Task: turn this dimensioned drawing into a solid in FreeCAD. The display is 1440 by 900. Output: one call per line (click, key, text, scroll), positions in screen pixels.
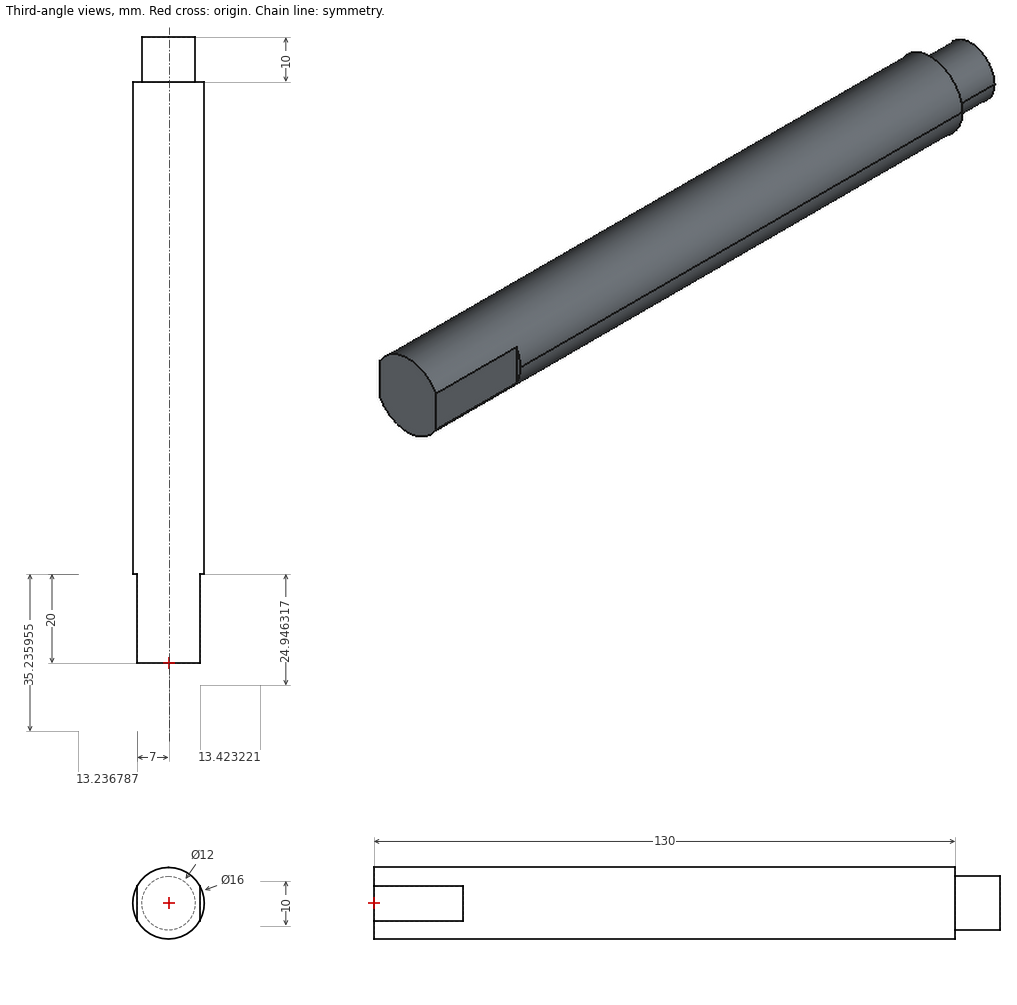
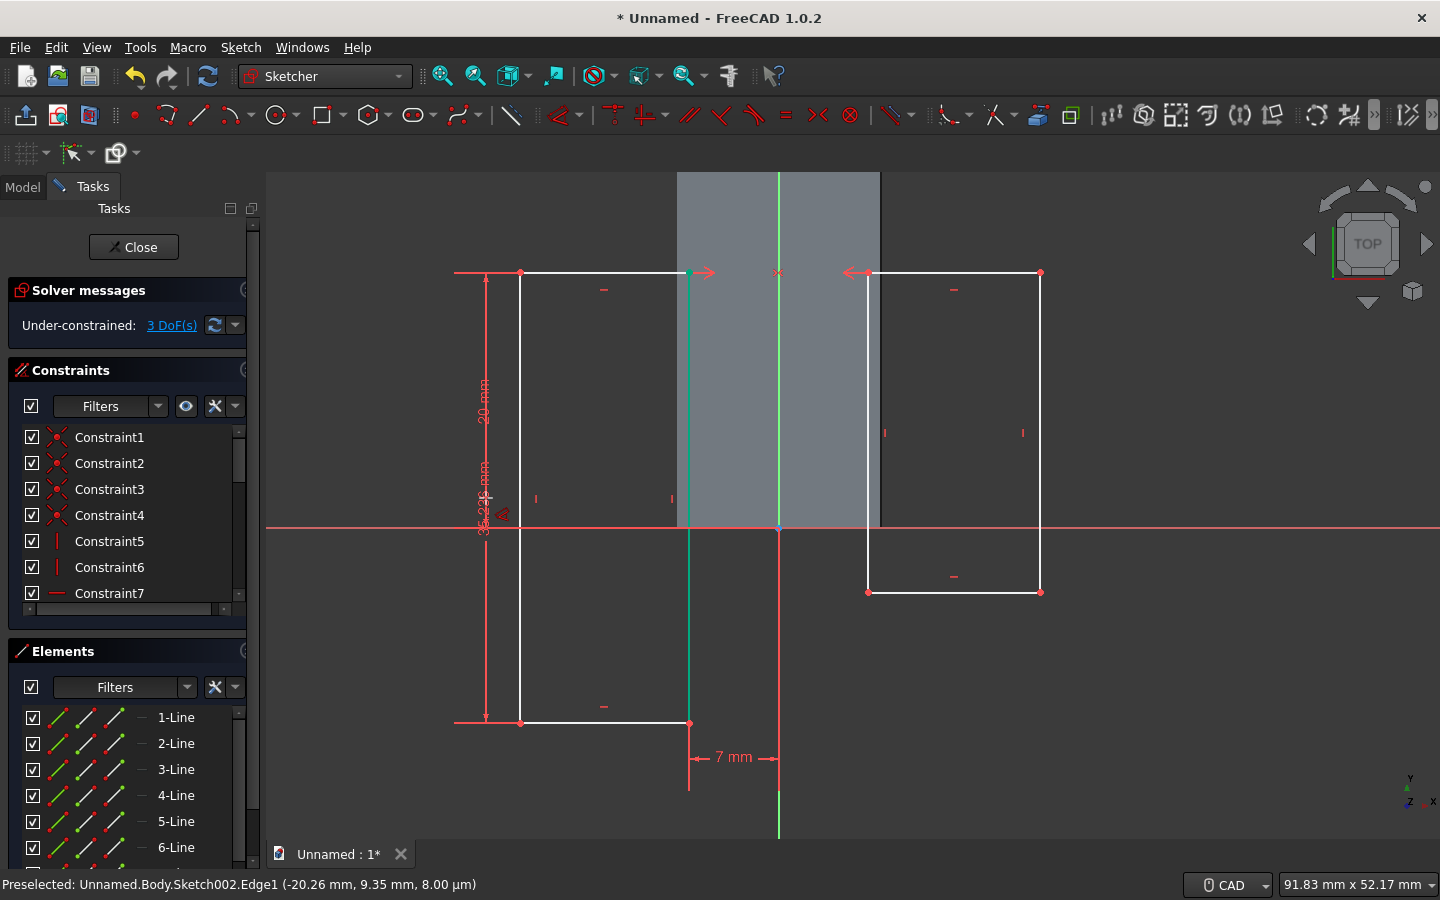
click(571, 723)
click(605, 757)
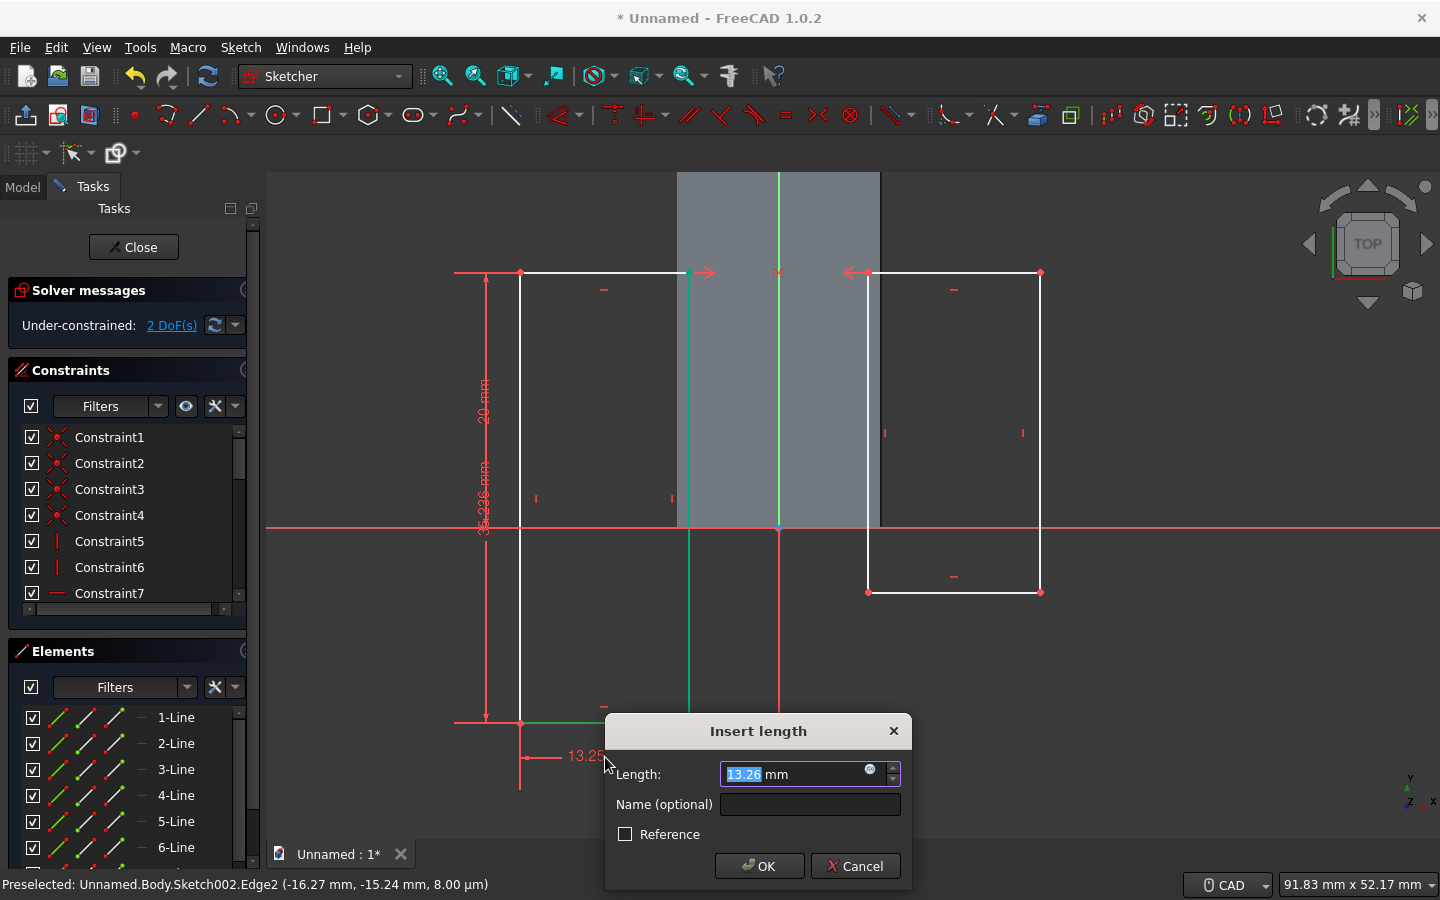
text(13.236787)
key(Return)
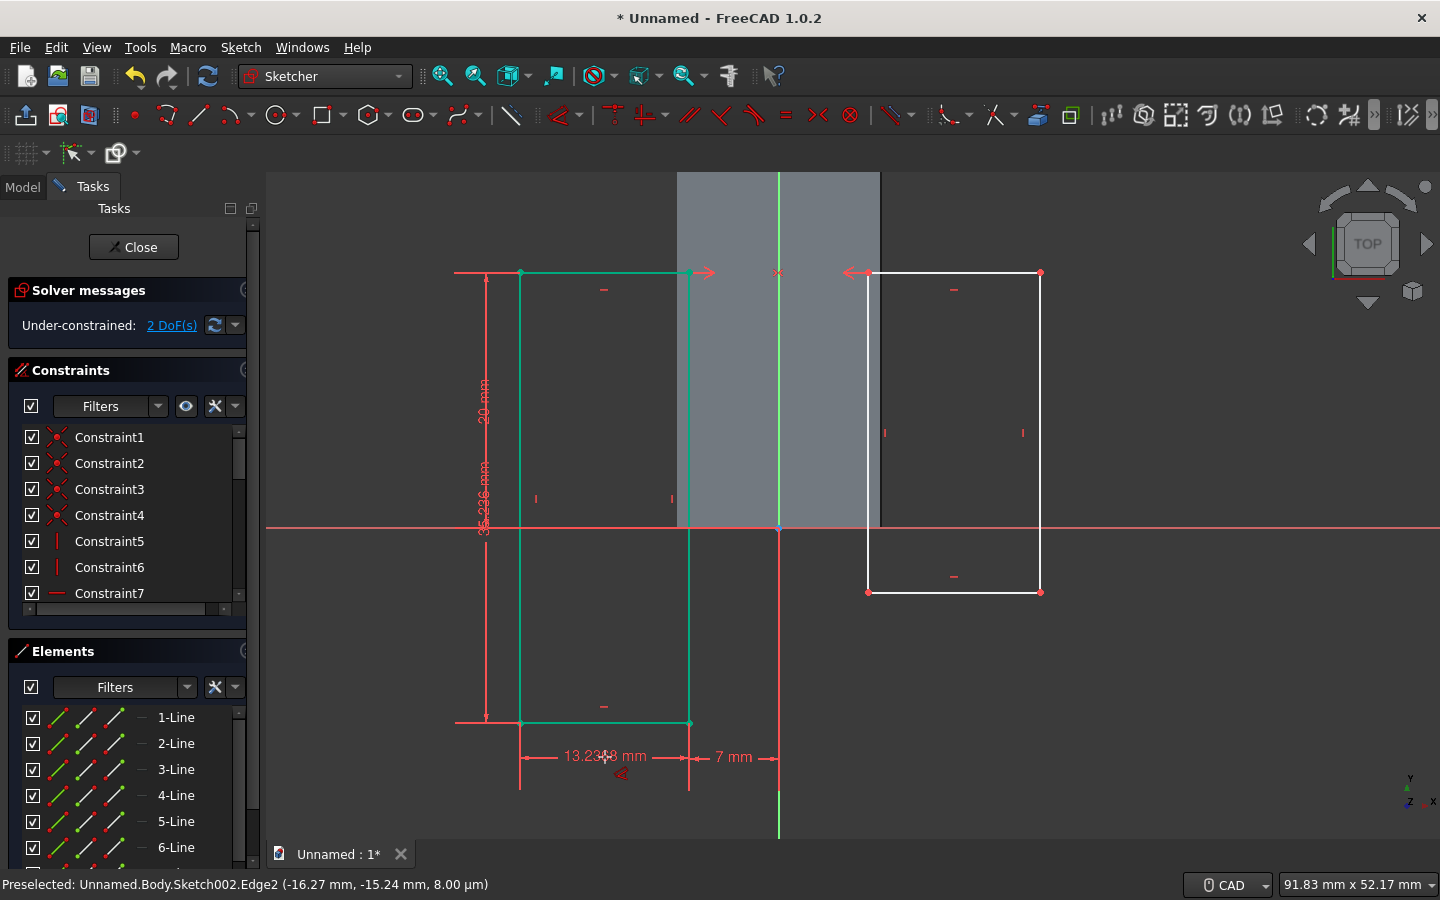
click(868, 369)
click(902, 433)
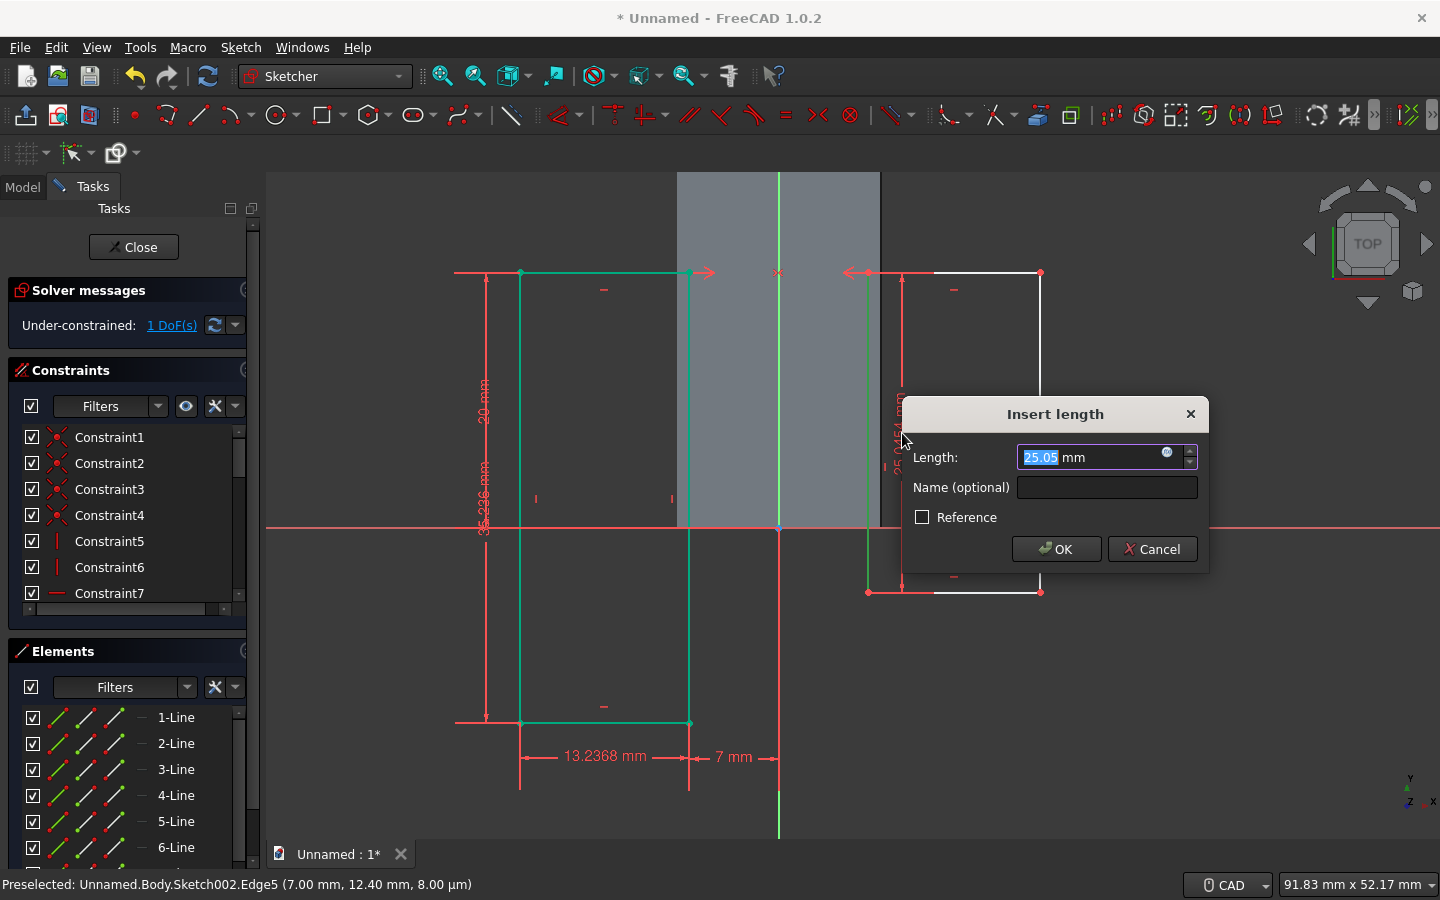
text(24.946317)
key(Return)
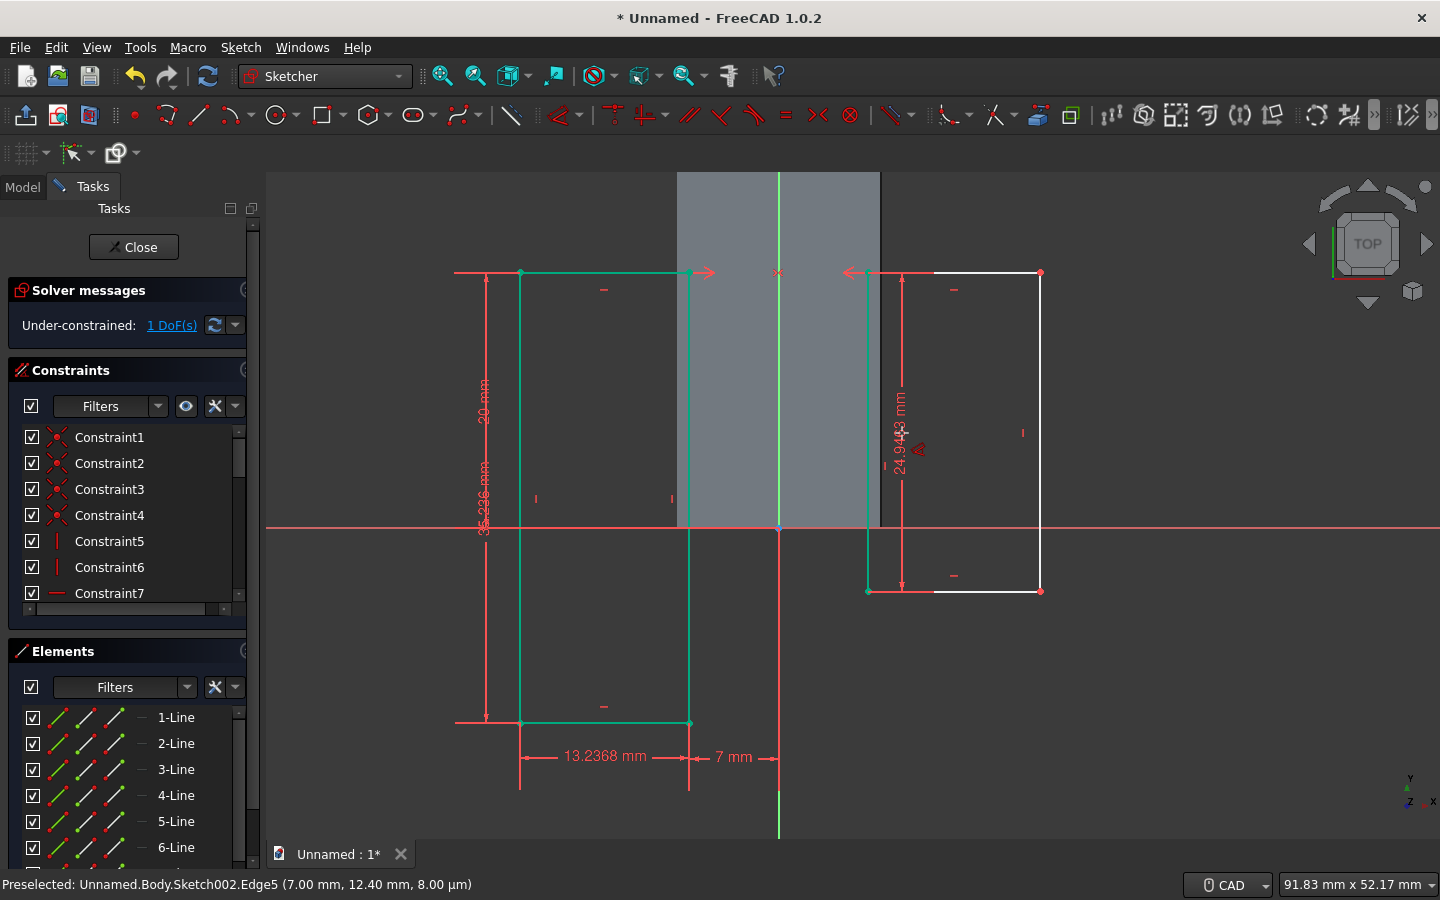
click(920, 592)
click(954, 626)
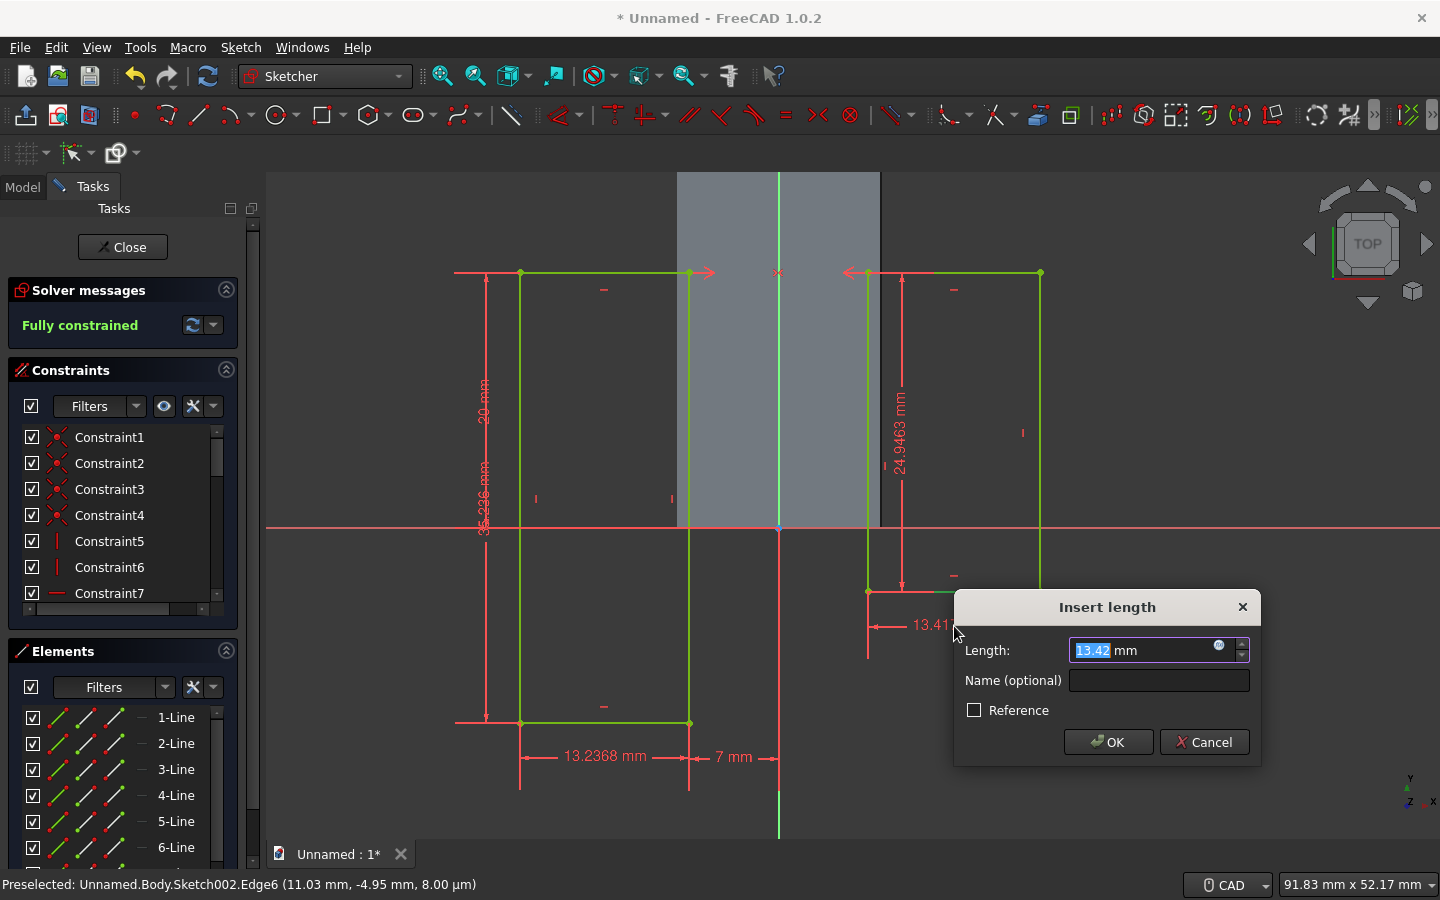
text(13.423221)
key(Return)
key(Escape)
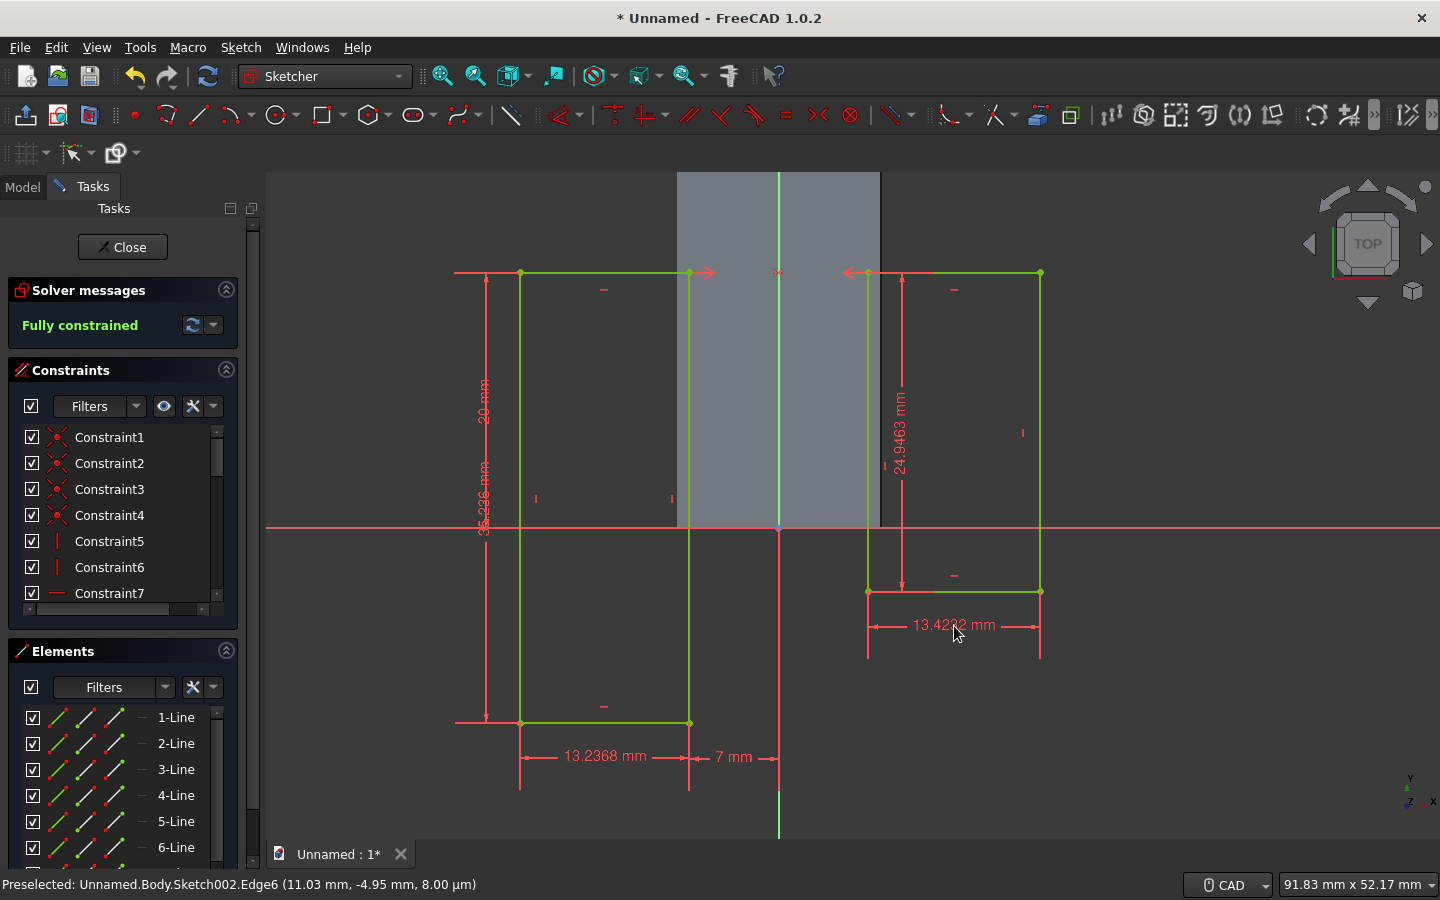
click(123, 247)